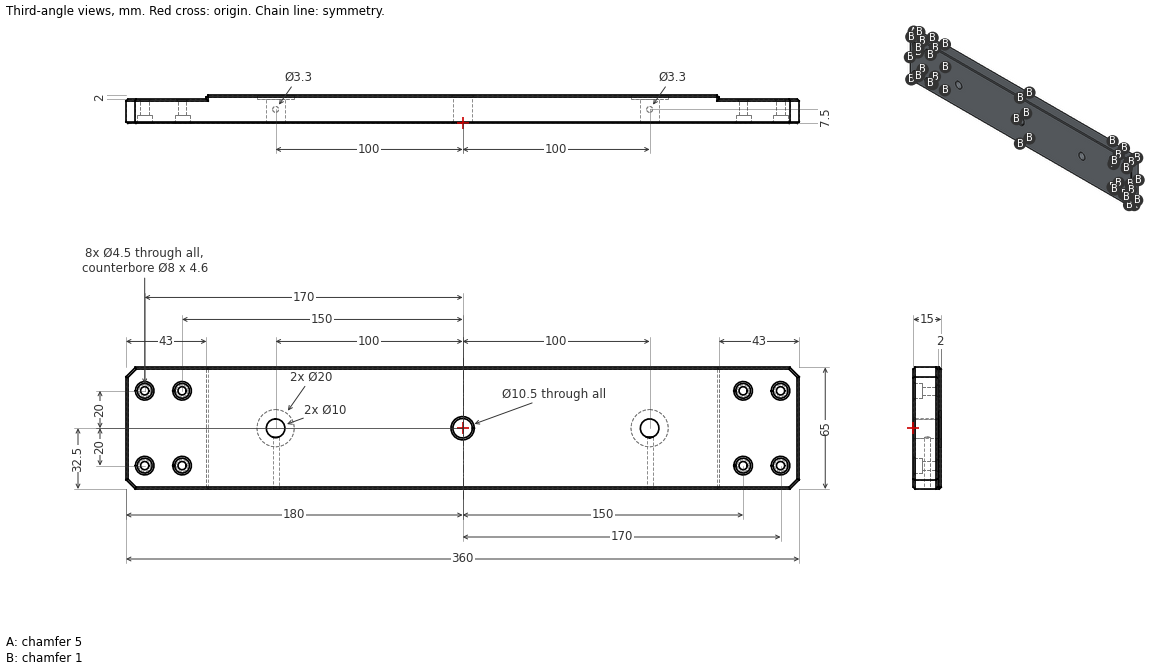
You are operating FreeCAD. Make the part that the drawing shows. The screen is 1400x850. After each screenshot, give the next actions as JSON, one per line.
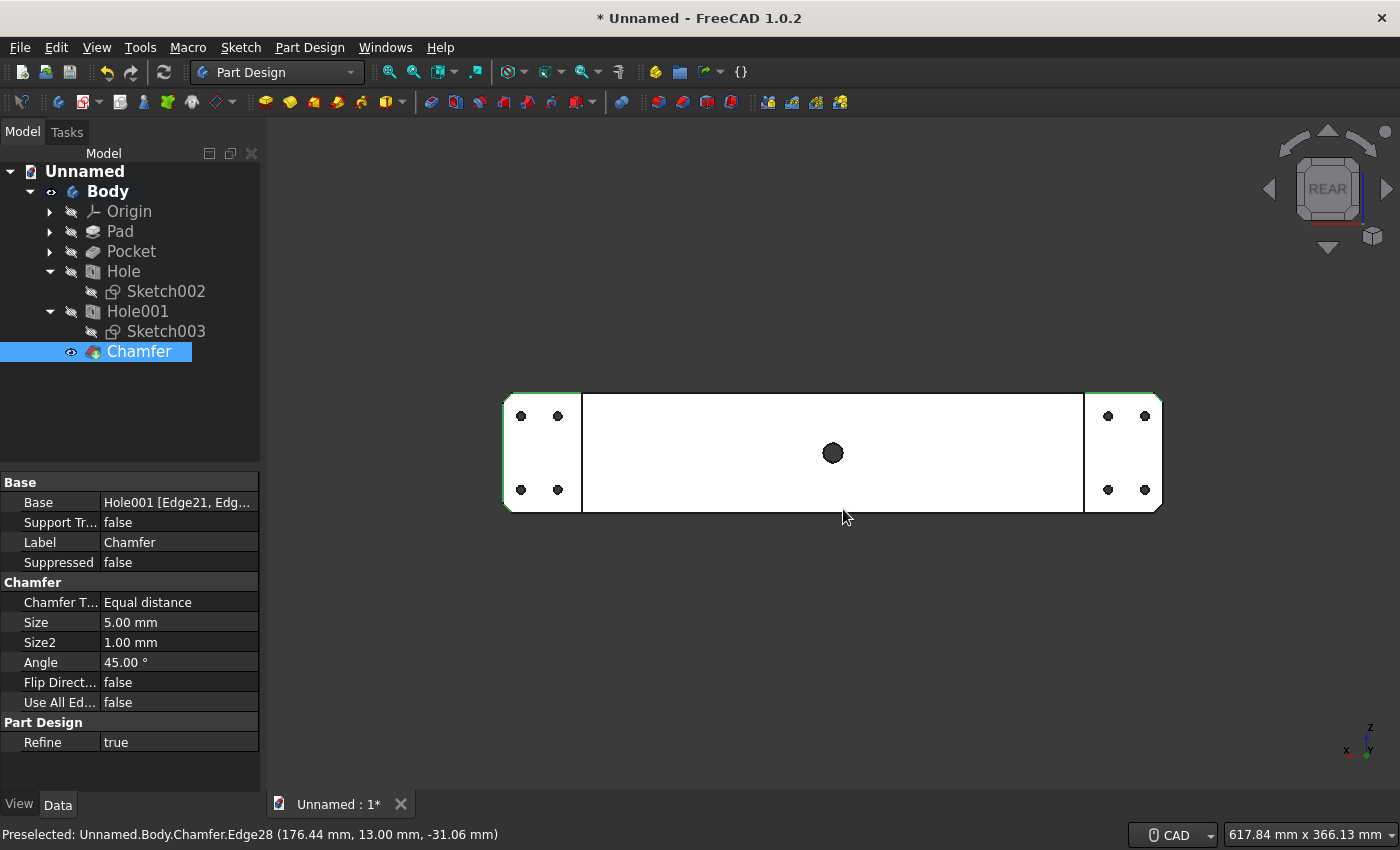
{"action": "left_click", "coordinate": [689, 452], "text": "ctrl"}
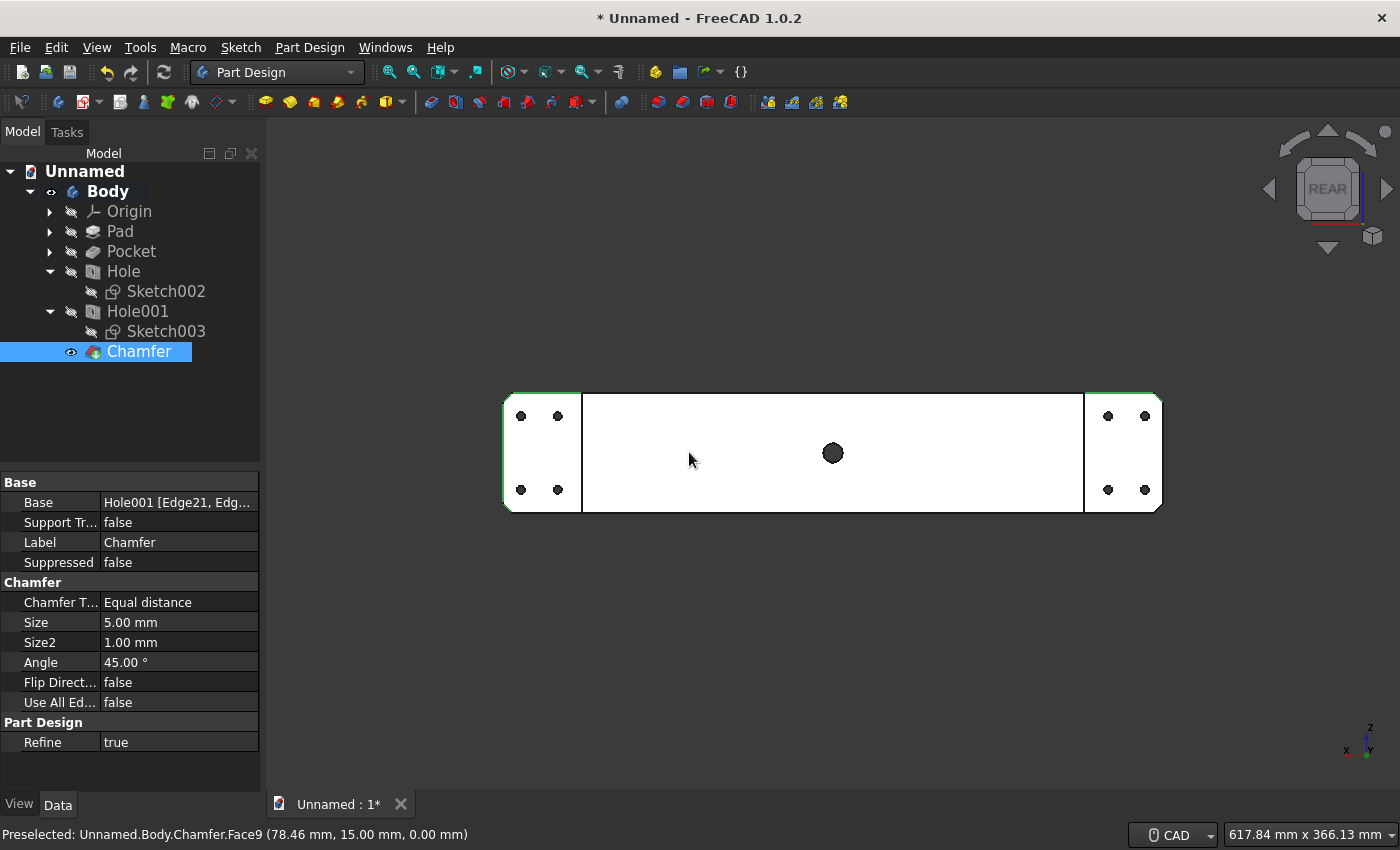
{"action": "left_click", "coordinate": [1163, 452], "text": "ctrl"}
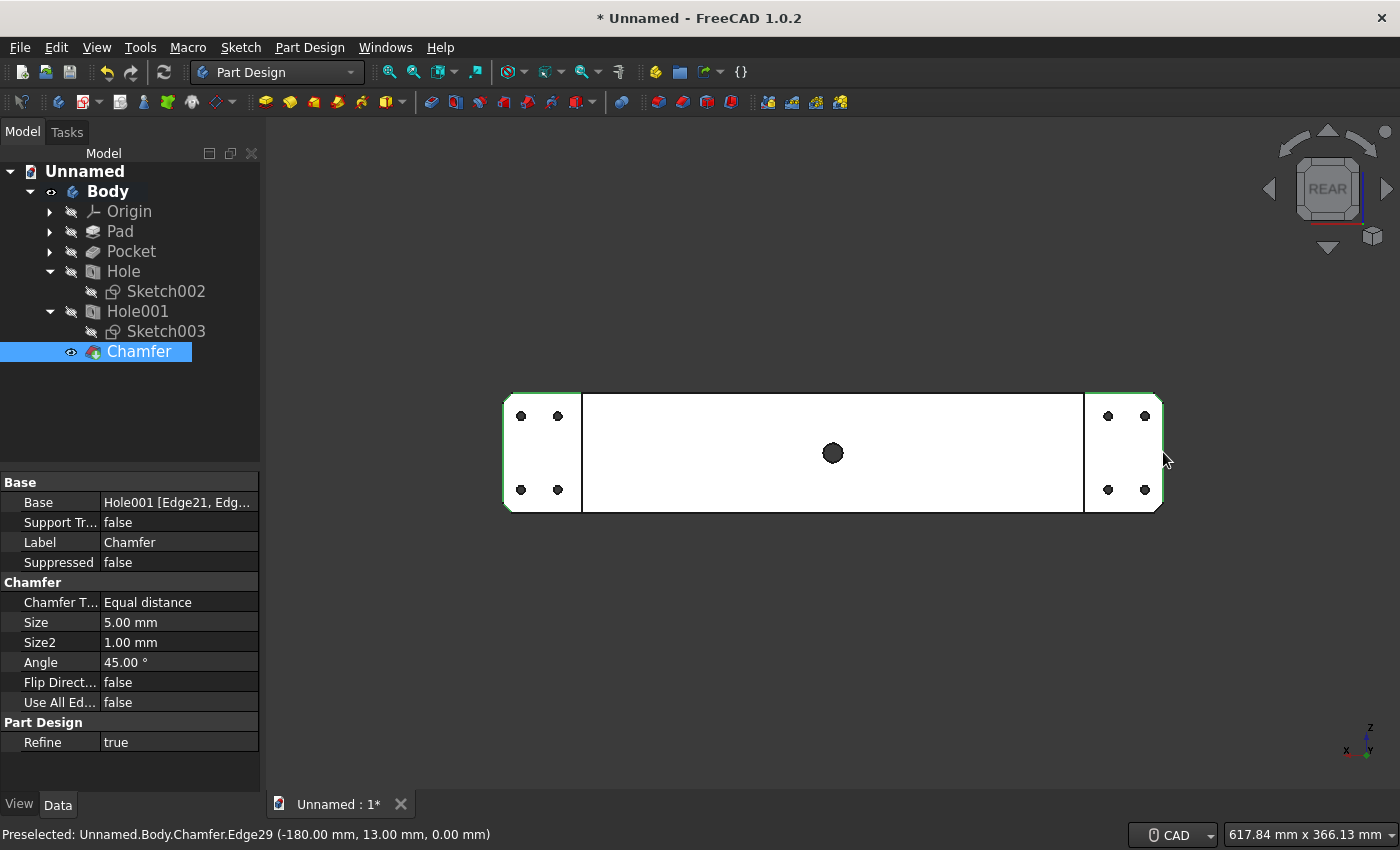
{"action": "left_click", "coordinate": [1159, 507], "text": "ctrl"}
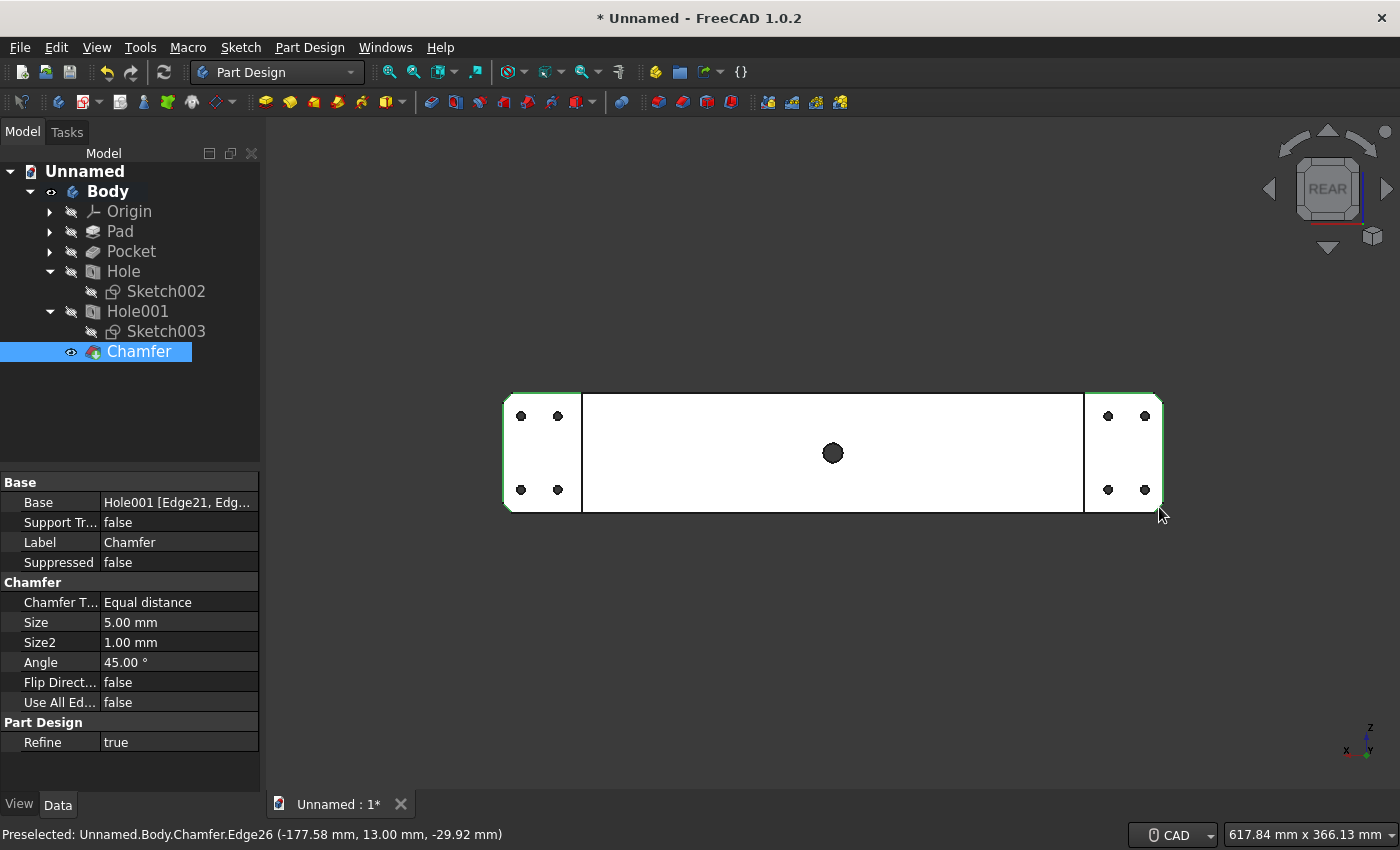
{"action": "left_click", "coordinate": [547, 512], "text": "ctrl"}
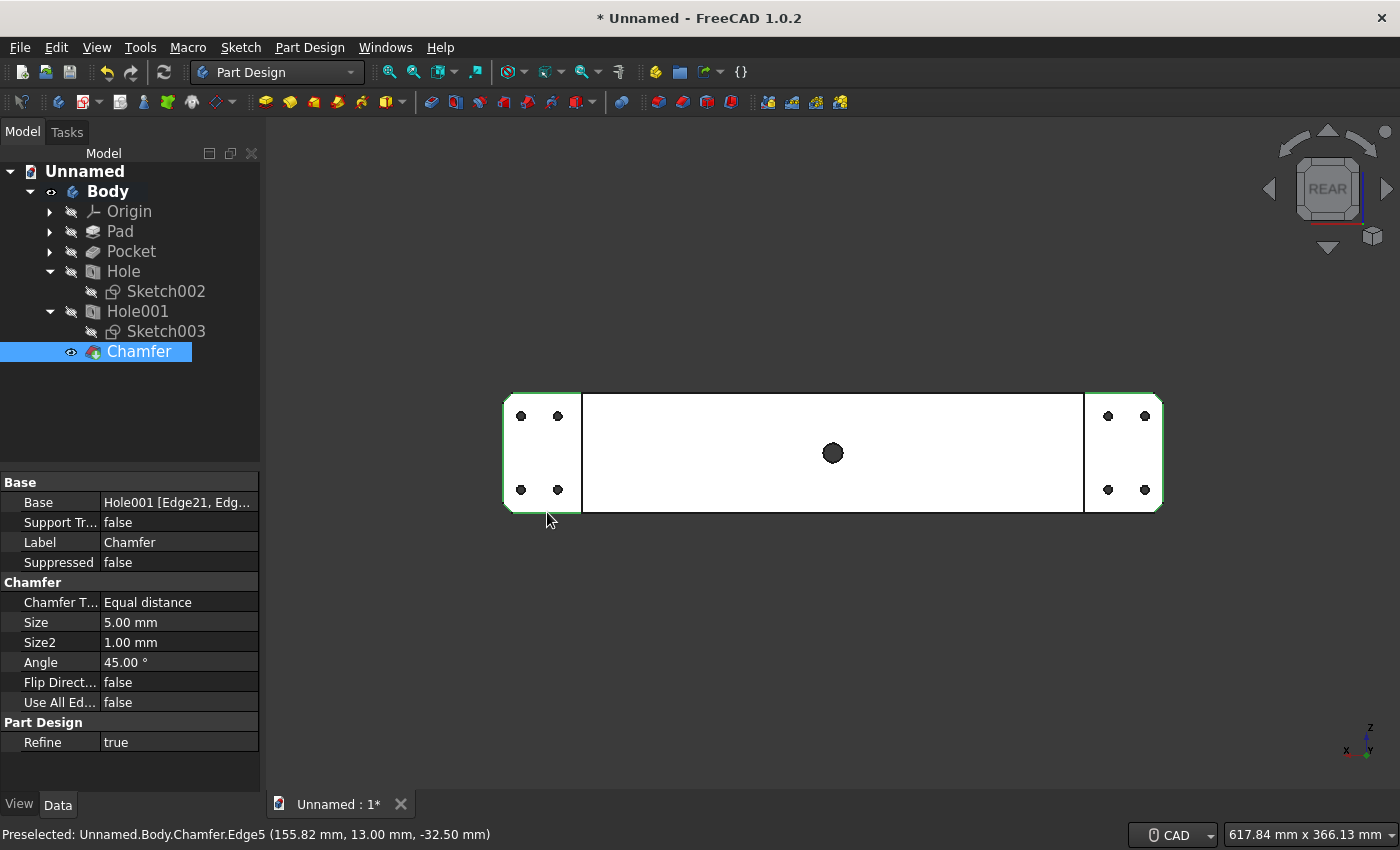
{"action": "left_click", "coordinate": [1119, 512], "text": "ctrl"}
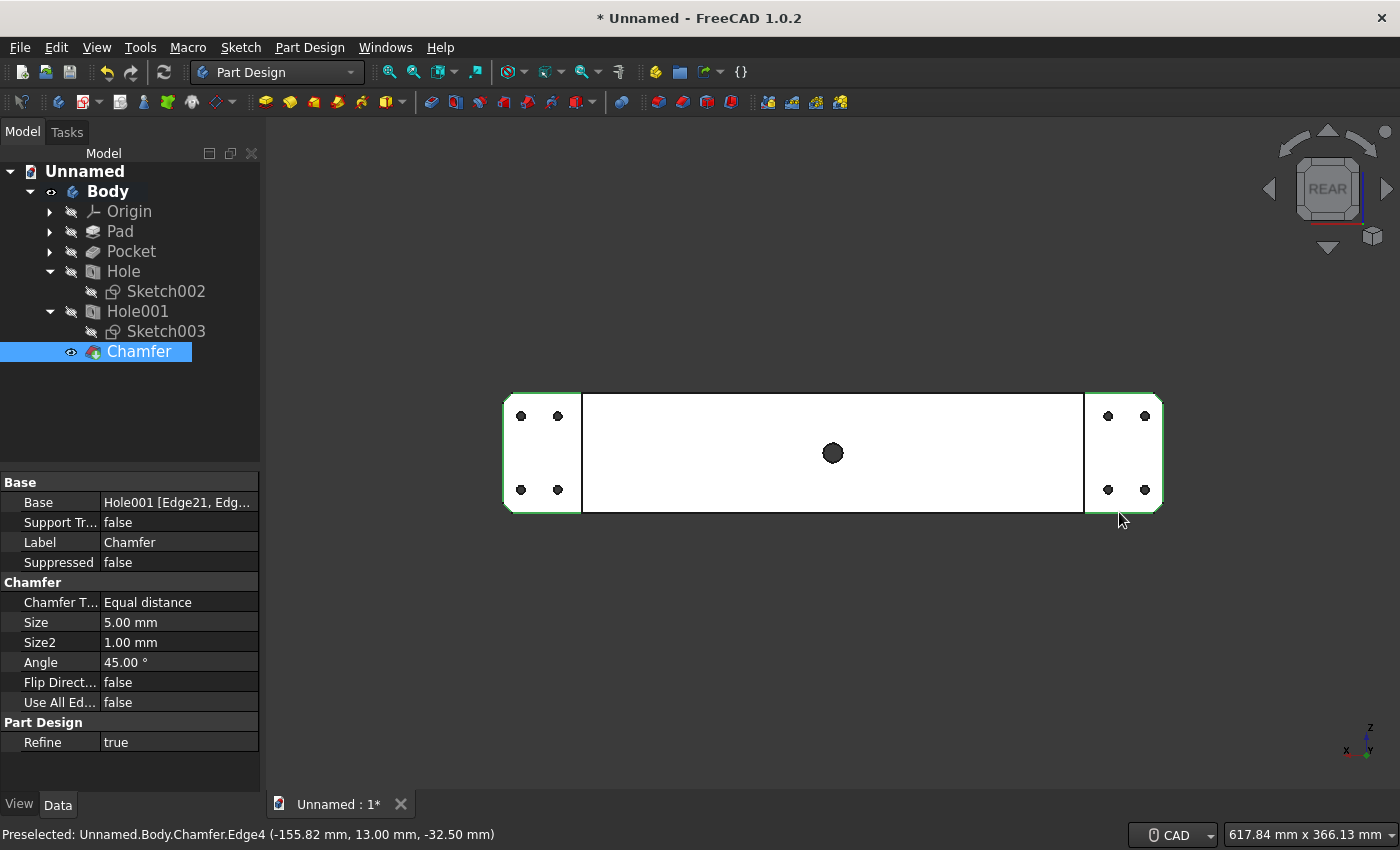
{"action": "left_click", "coordinate": [525, 415], "text": "ctrl"}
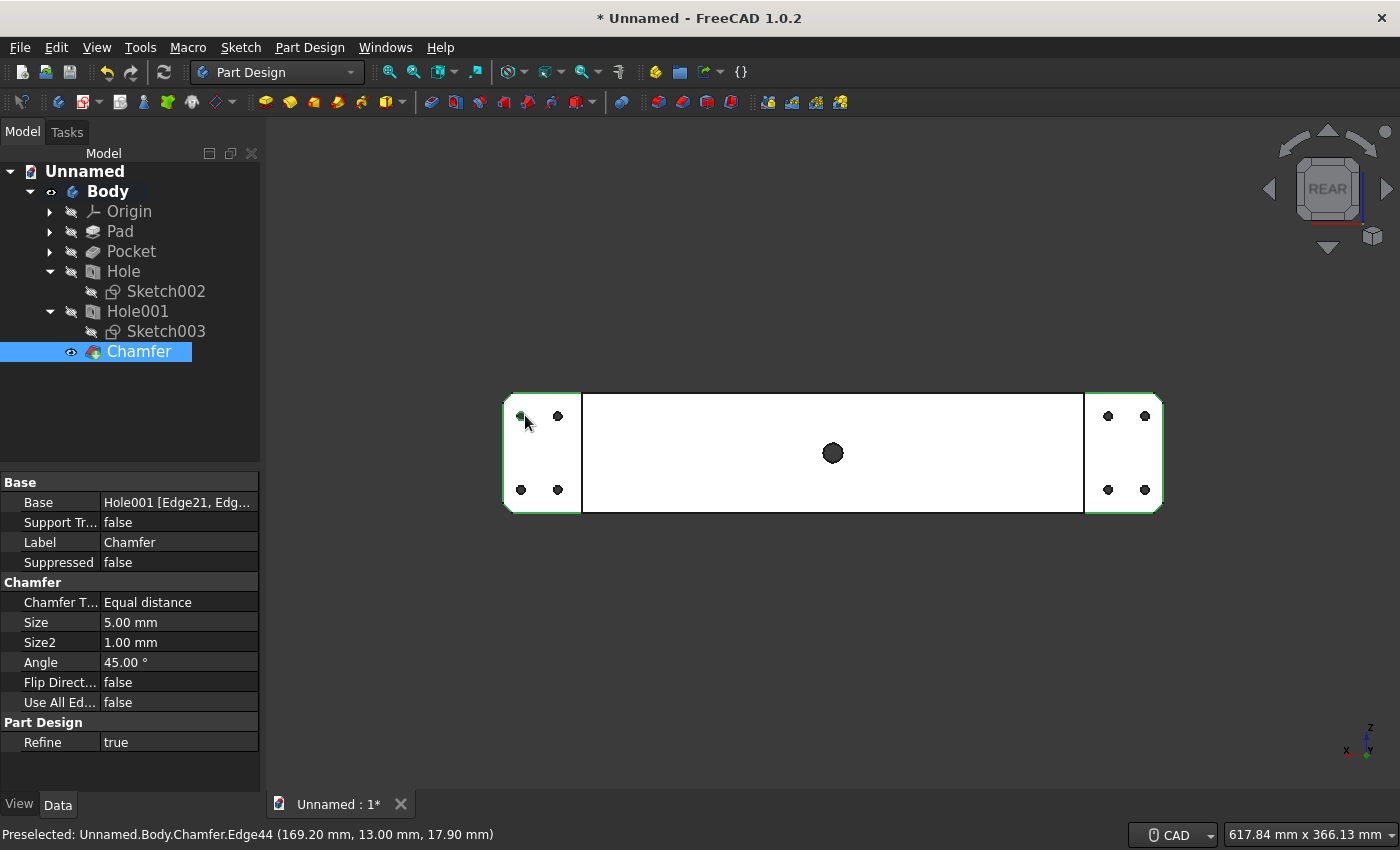
{"action": "left_click", "coordinate": [562, 415], "text": "ctrl"}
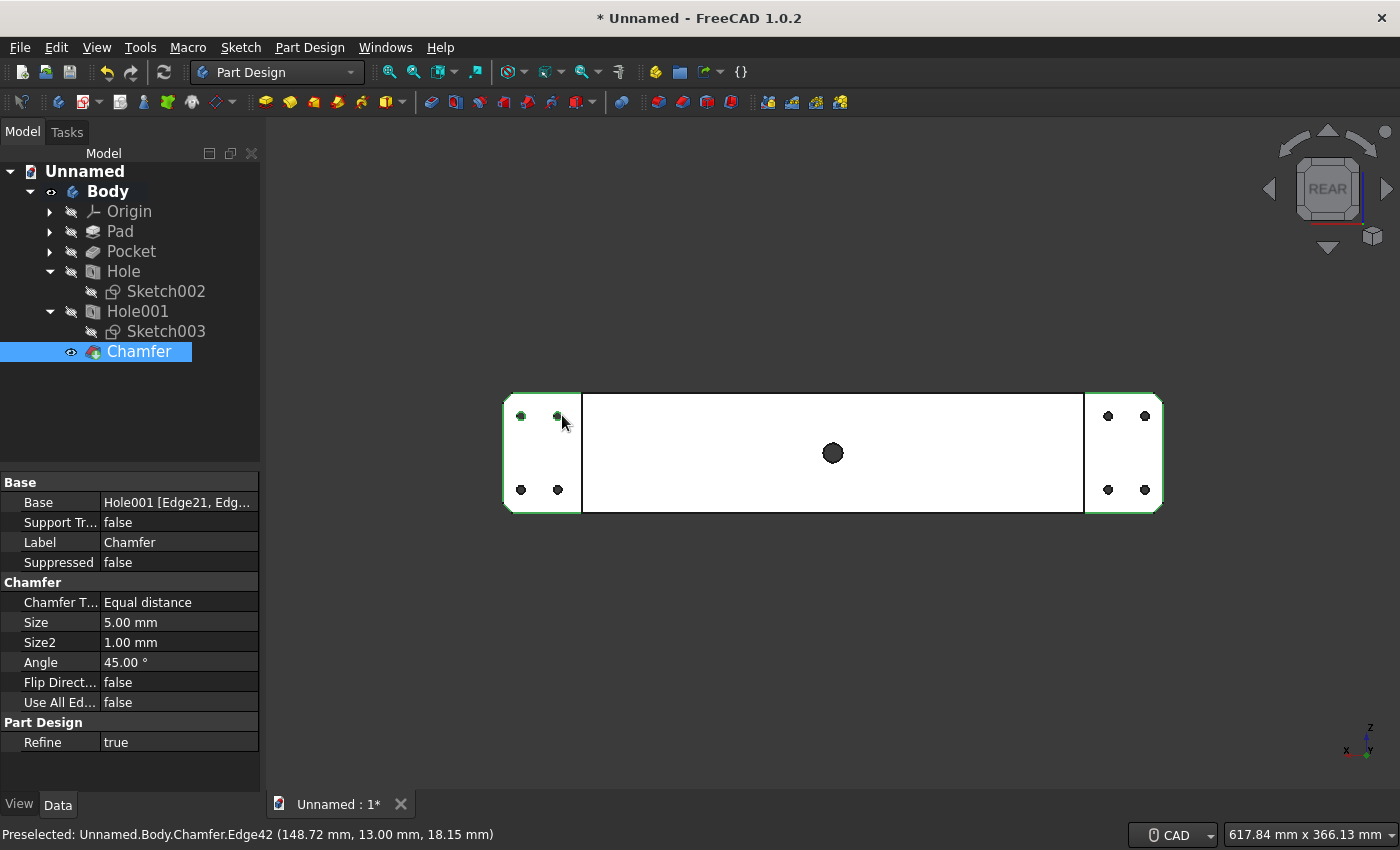
{"action": "left_click", "coordinate": [525, 489], "text": "ctrl"}